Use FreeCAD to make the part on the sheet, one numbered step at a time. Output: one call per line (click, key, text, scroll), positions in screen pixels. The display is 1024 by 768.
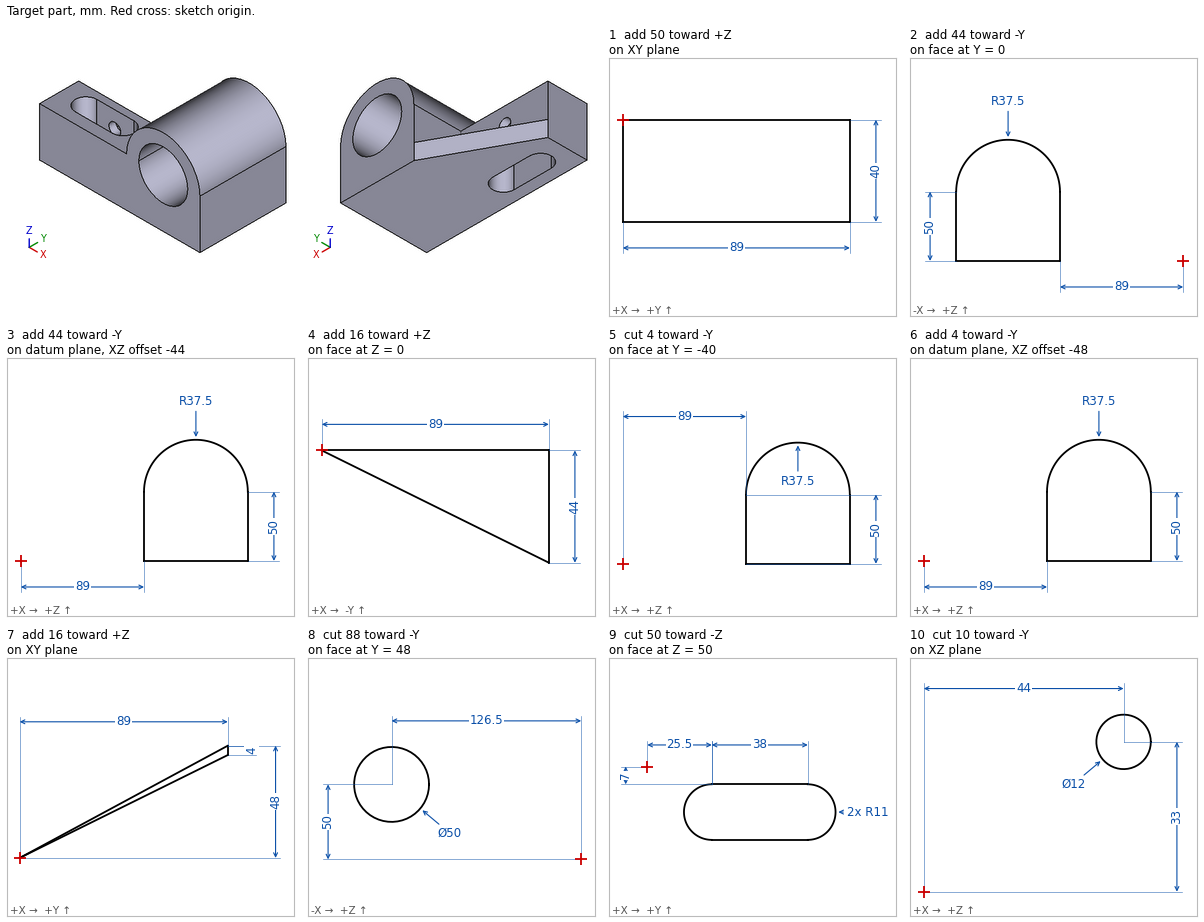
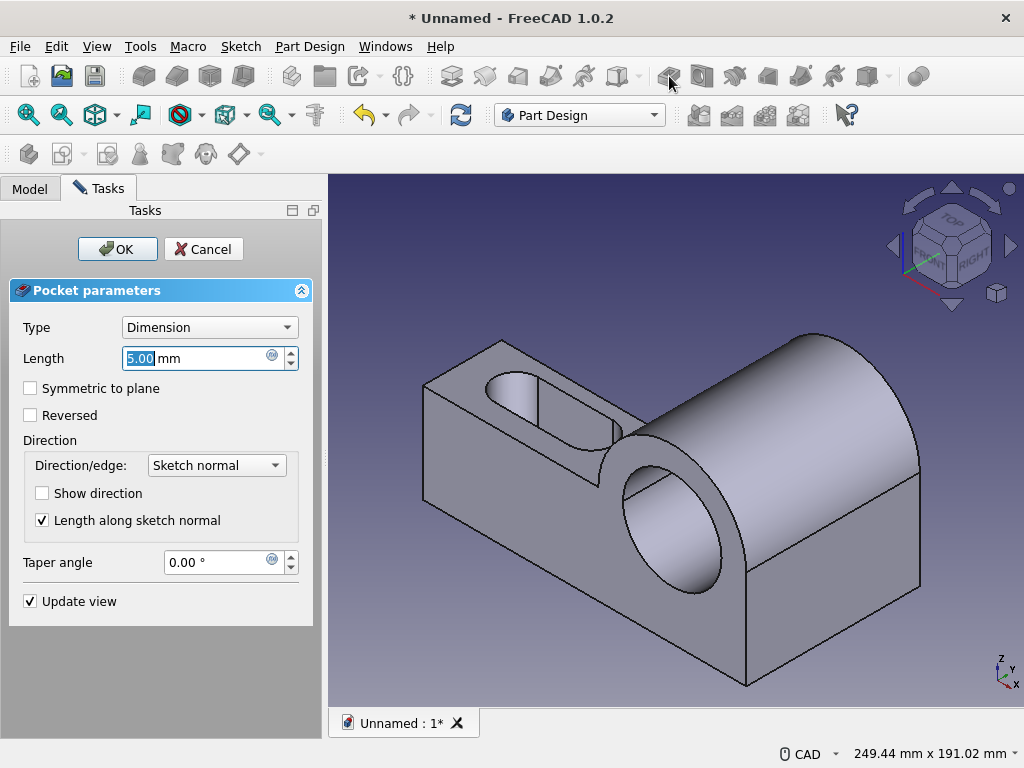
text(10)
key(Tab)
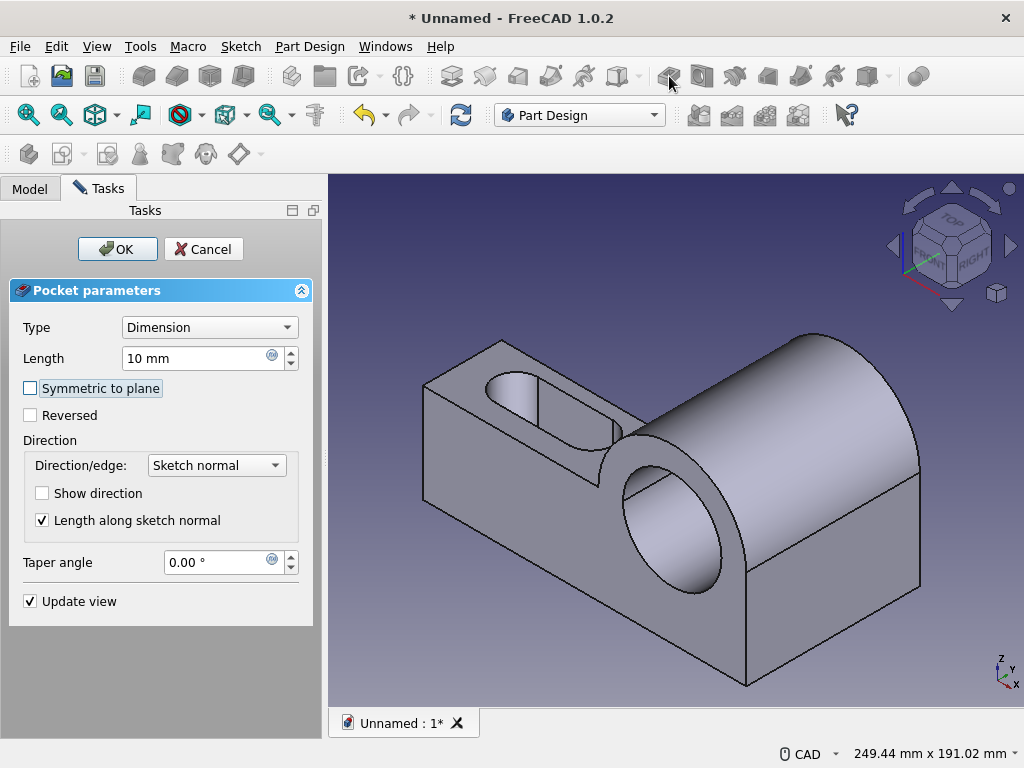
click(31, 415)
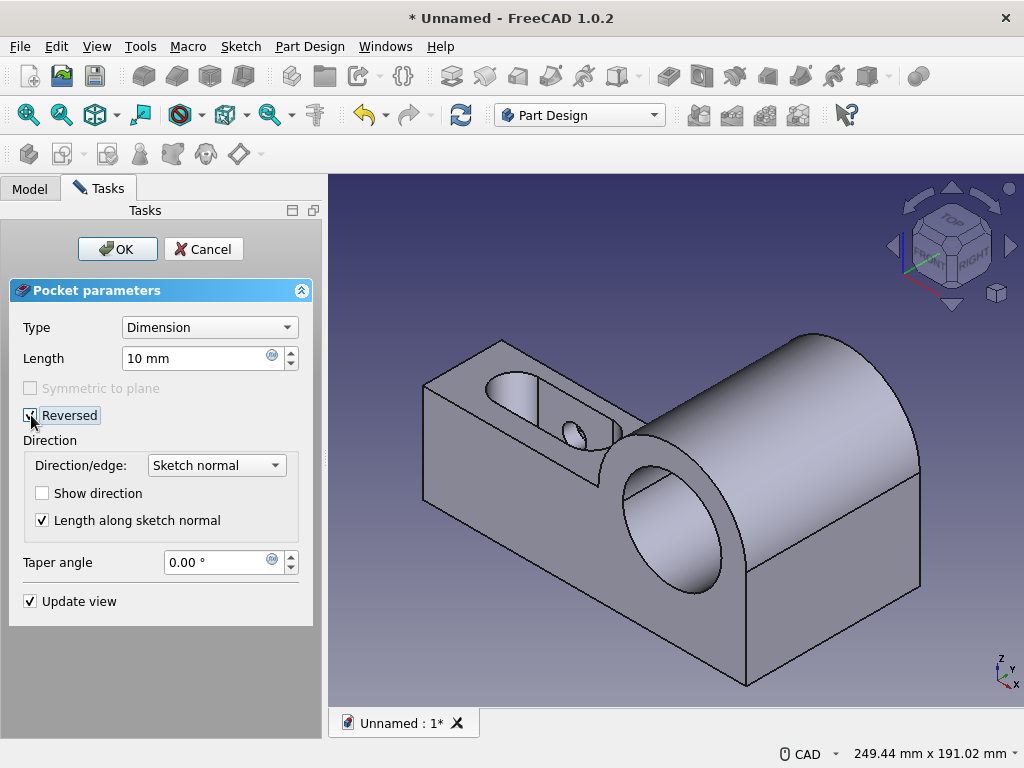
click(118, 249)